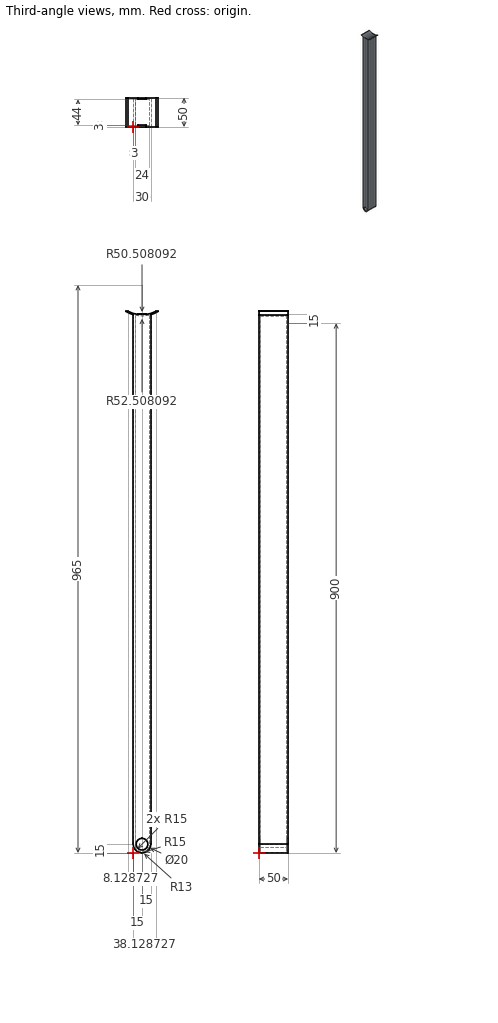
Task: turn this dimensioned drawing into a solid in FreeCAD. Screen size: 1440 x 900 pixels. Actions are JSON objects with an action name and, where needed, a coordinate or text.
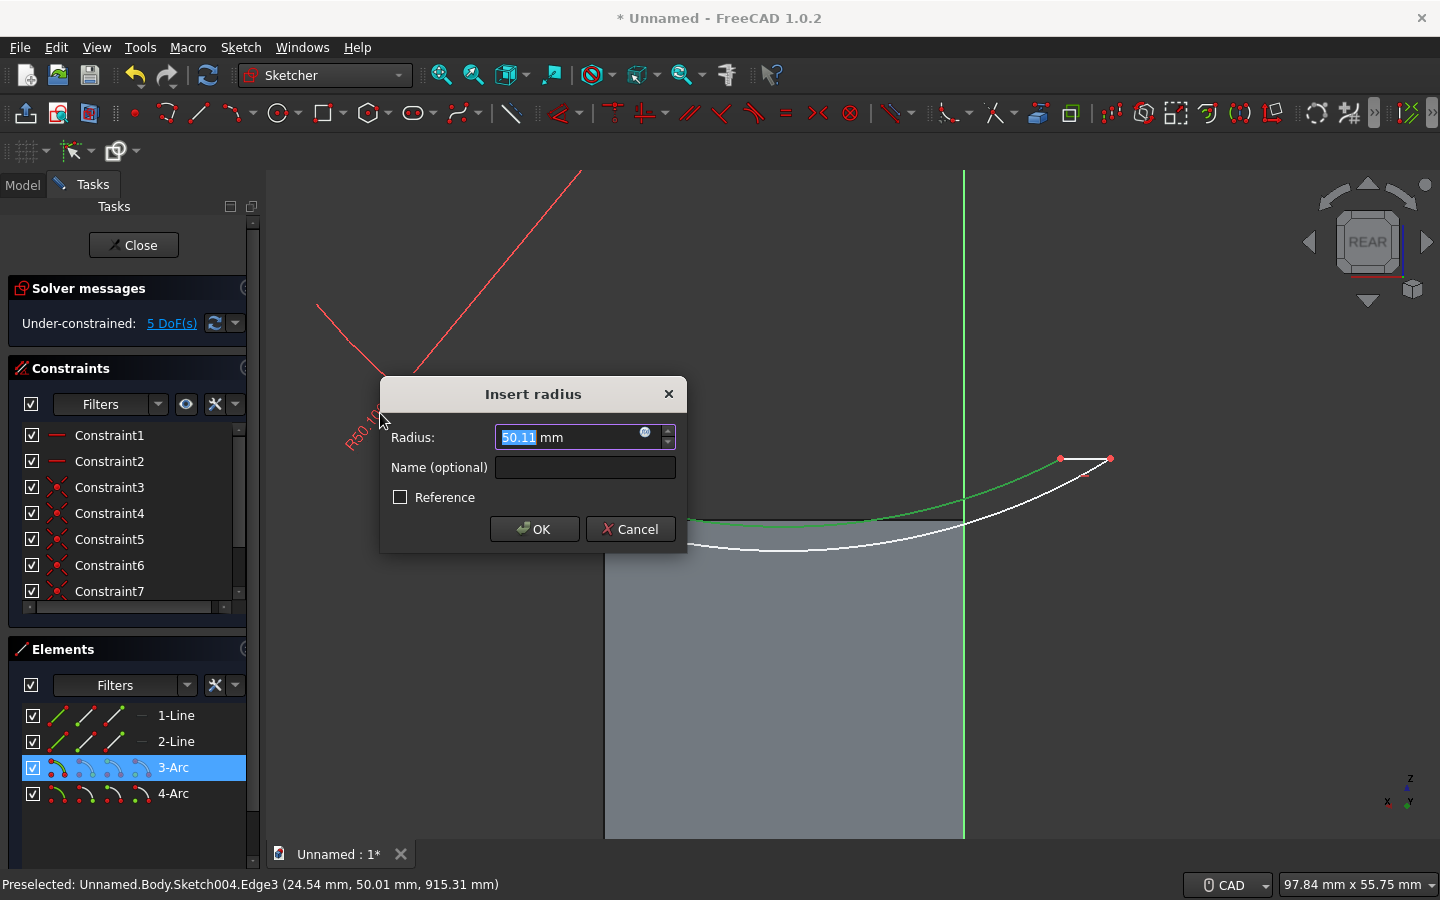
{"action": "type", "text": "50.508092"}
{"action": "key", "text": "Return"}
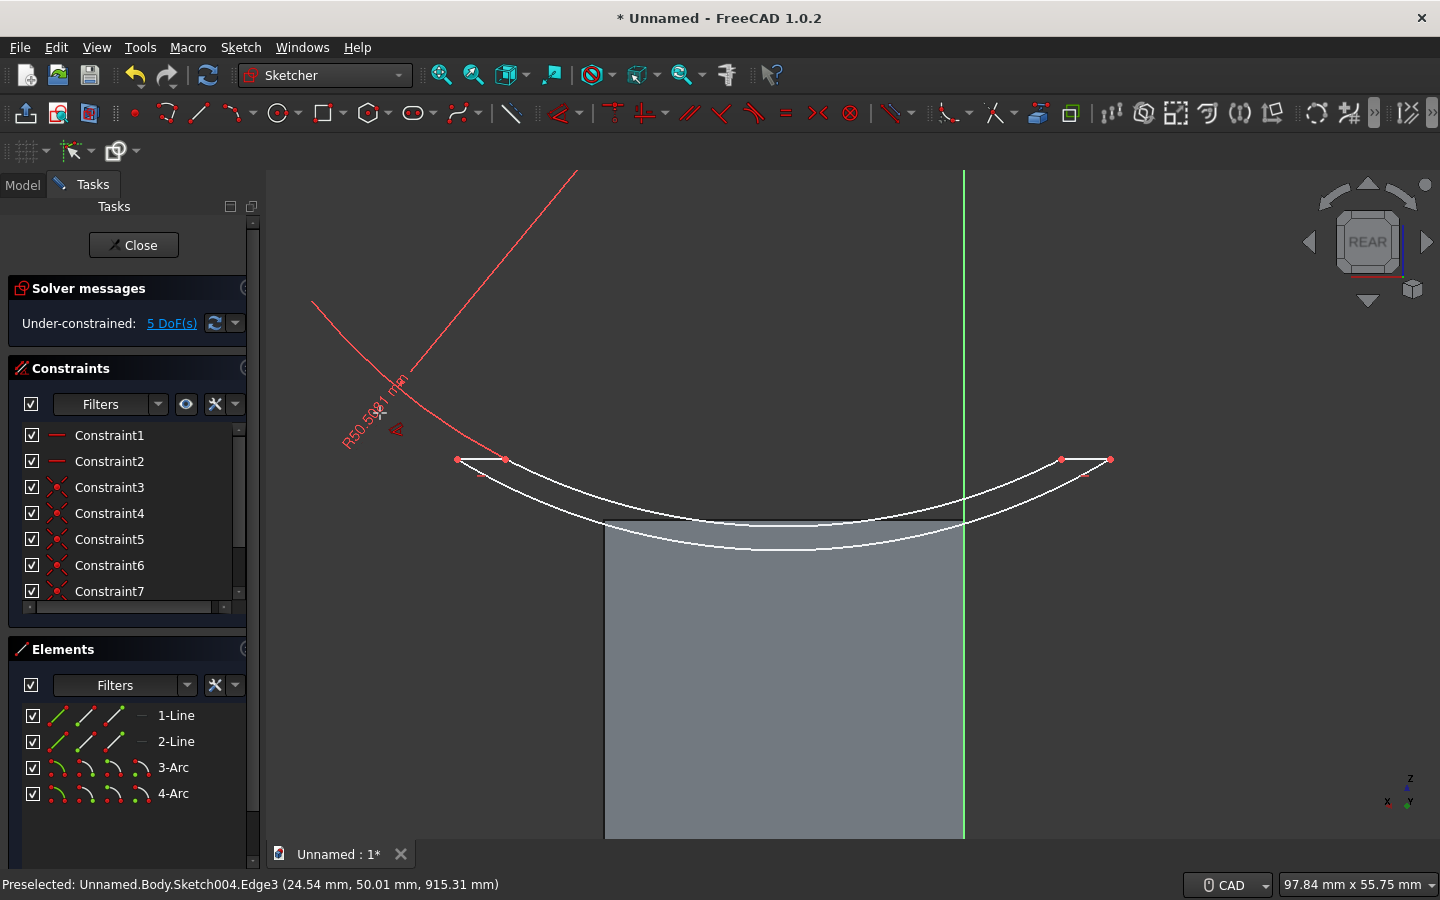
{"action": "left_click", "coordinate": [647, 535]}
{"action": "left_click", "coordinate": [640, 566]}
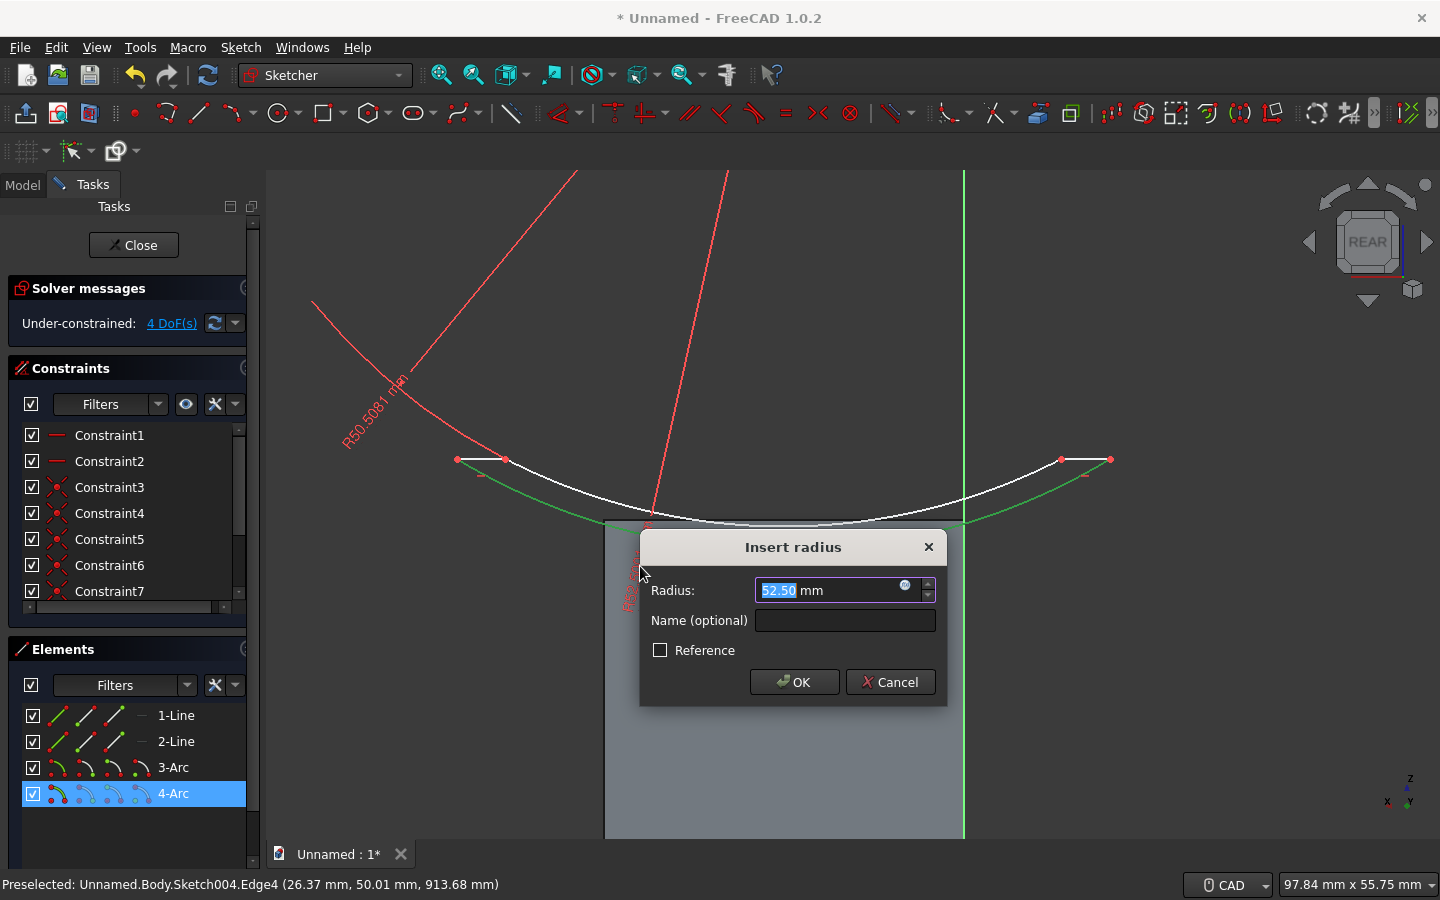
{"action": "type", "text": "52.508092"}
{"action": "key", "text": "Return"}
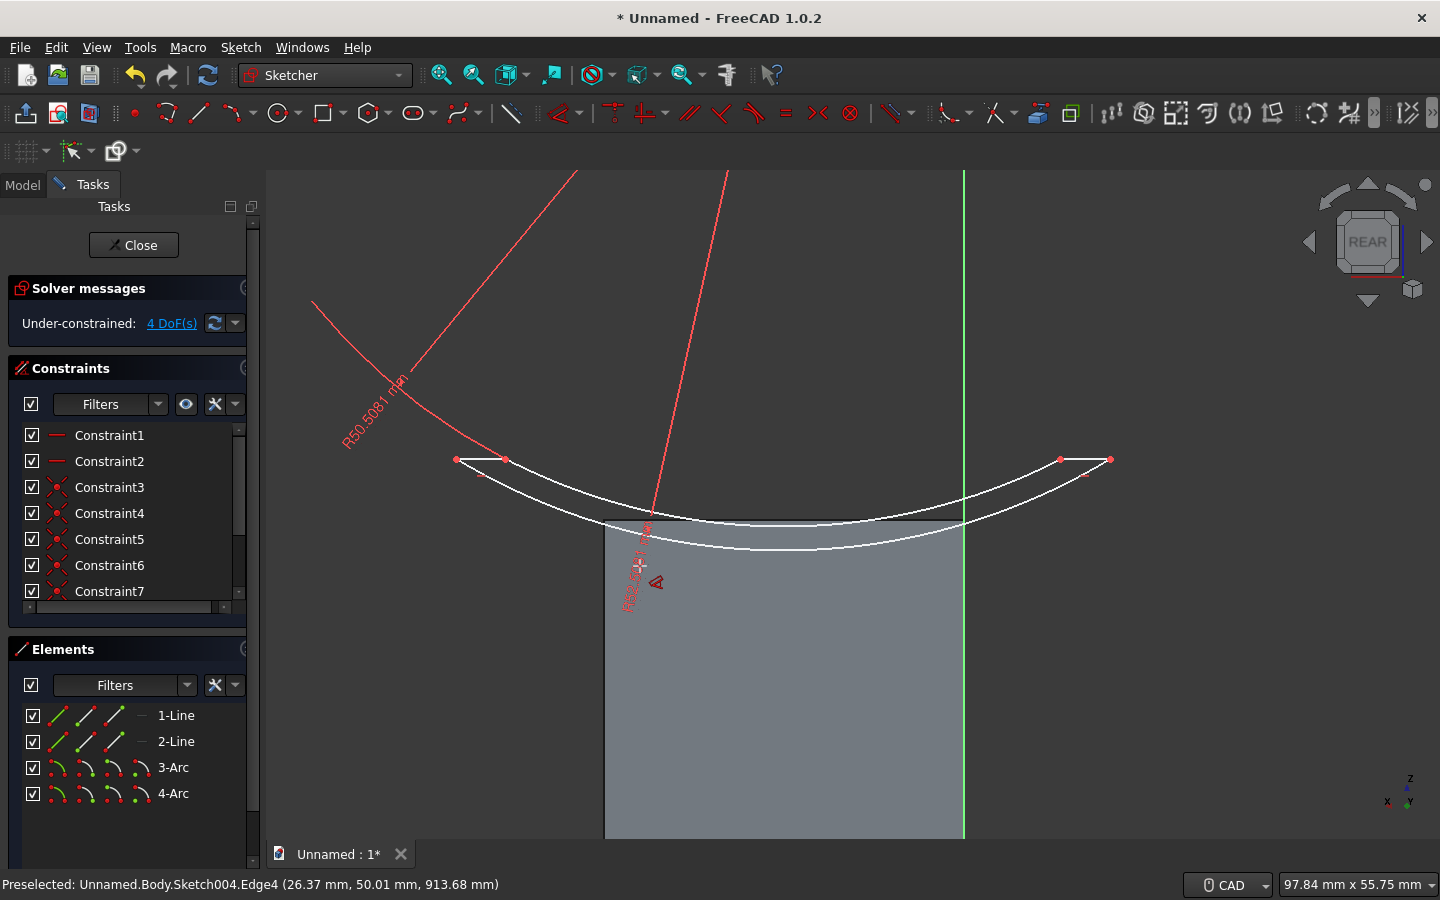
{"action": "scroll", "coordinate": [786, 811], "scroll_direction": "down", "scroll_amount": 3}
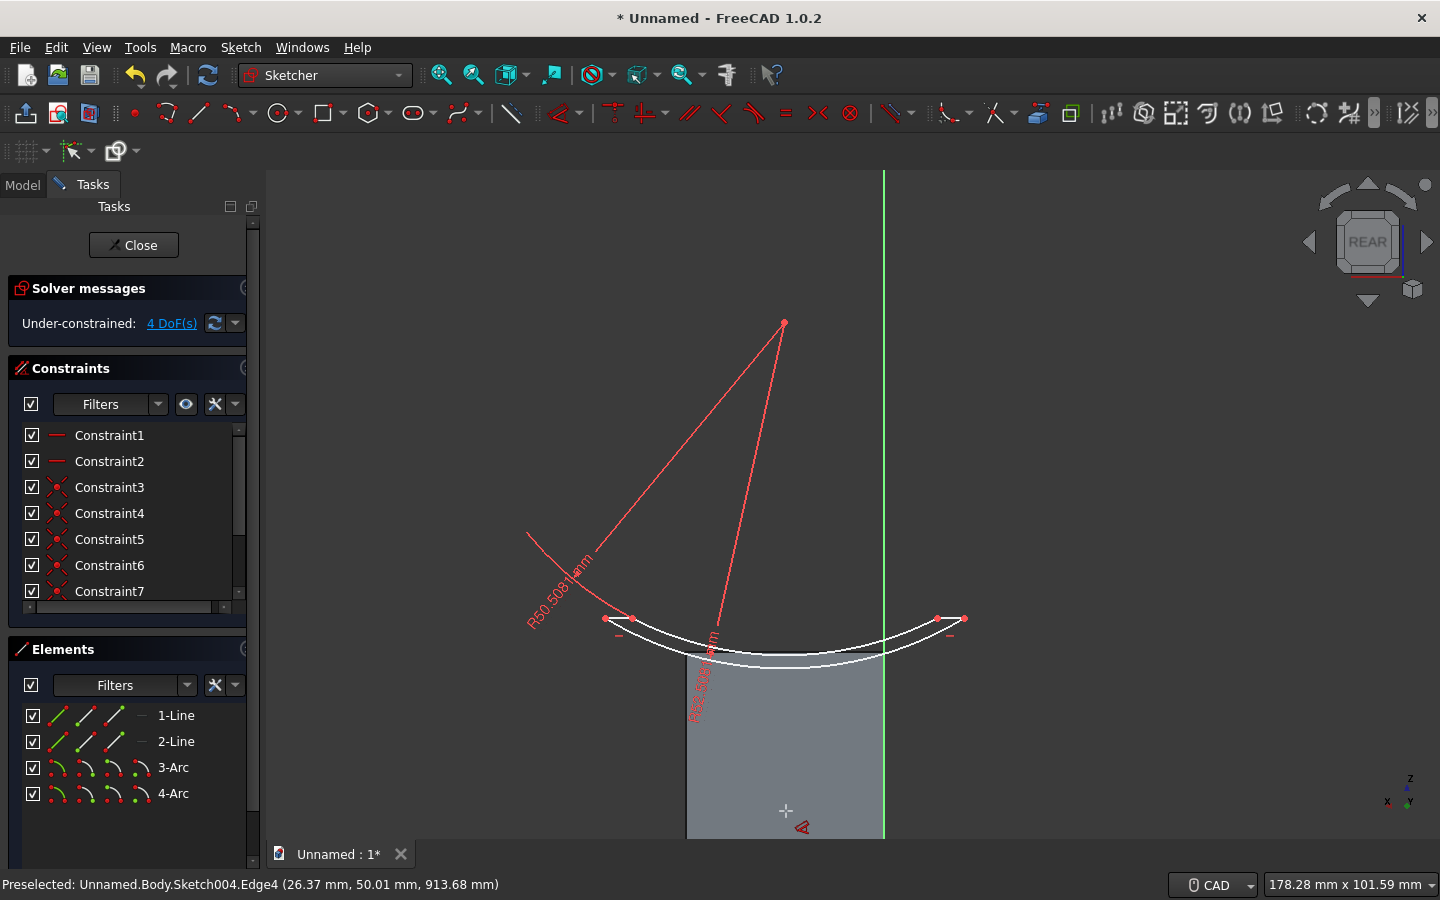
{"action": "left_click", "coordinate": [785, 323]}
{"action": "left_click", "coordinate": [834, 289]}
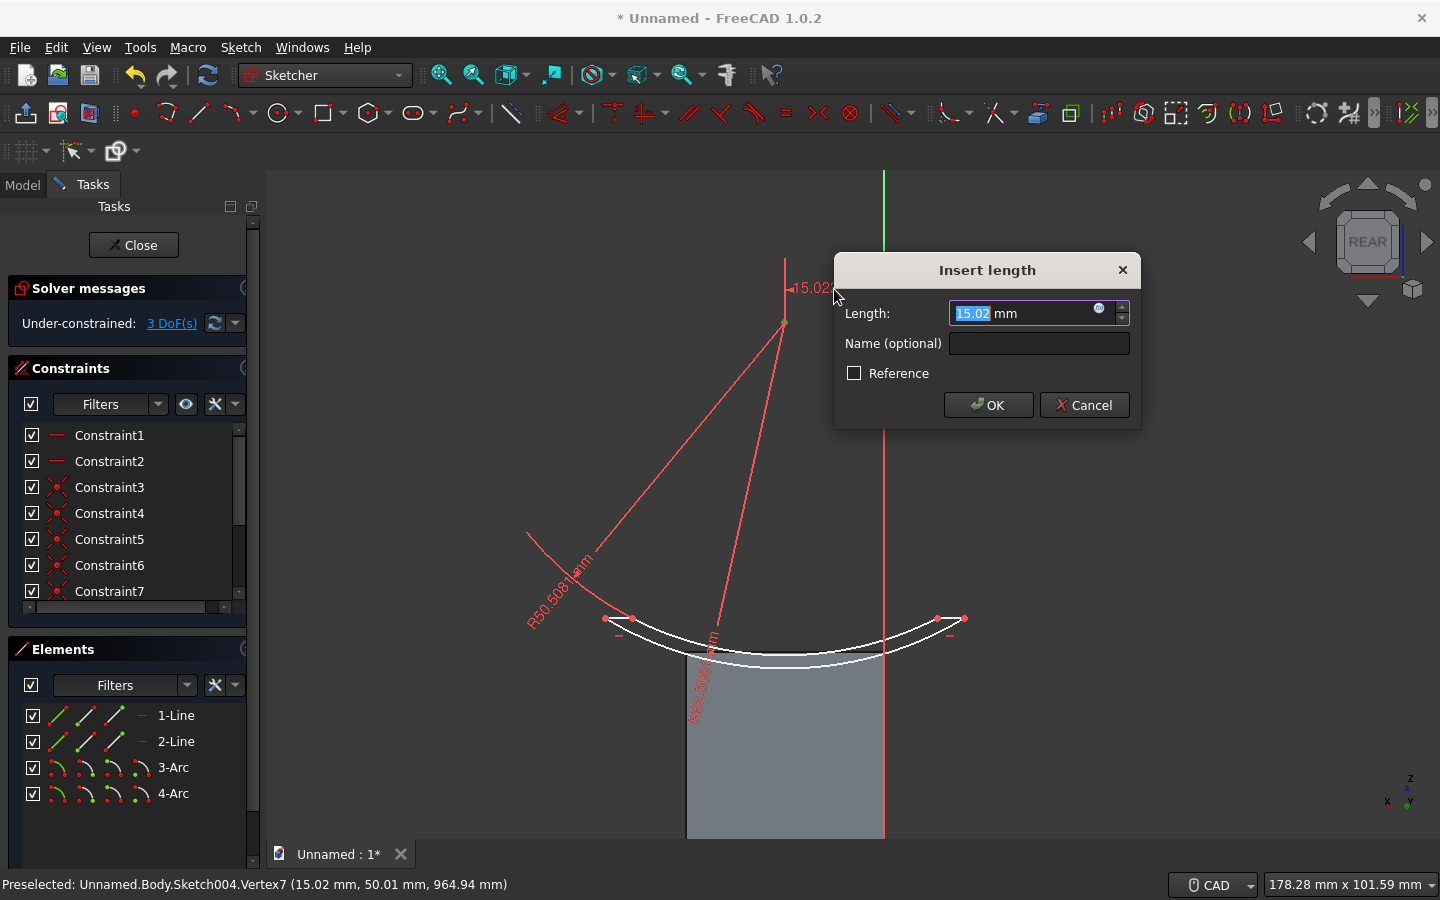
{"action": "type", "text": "15"}
{"action": "key", "text": "Return"}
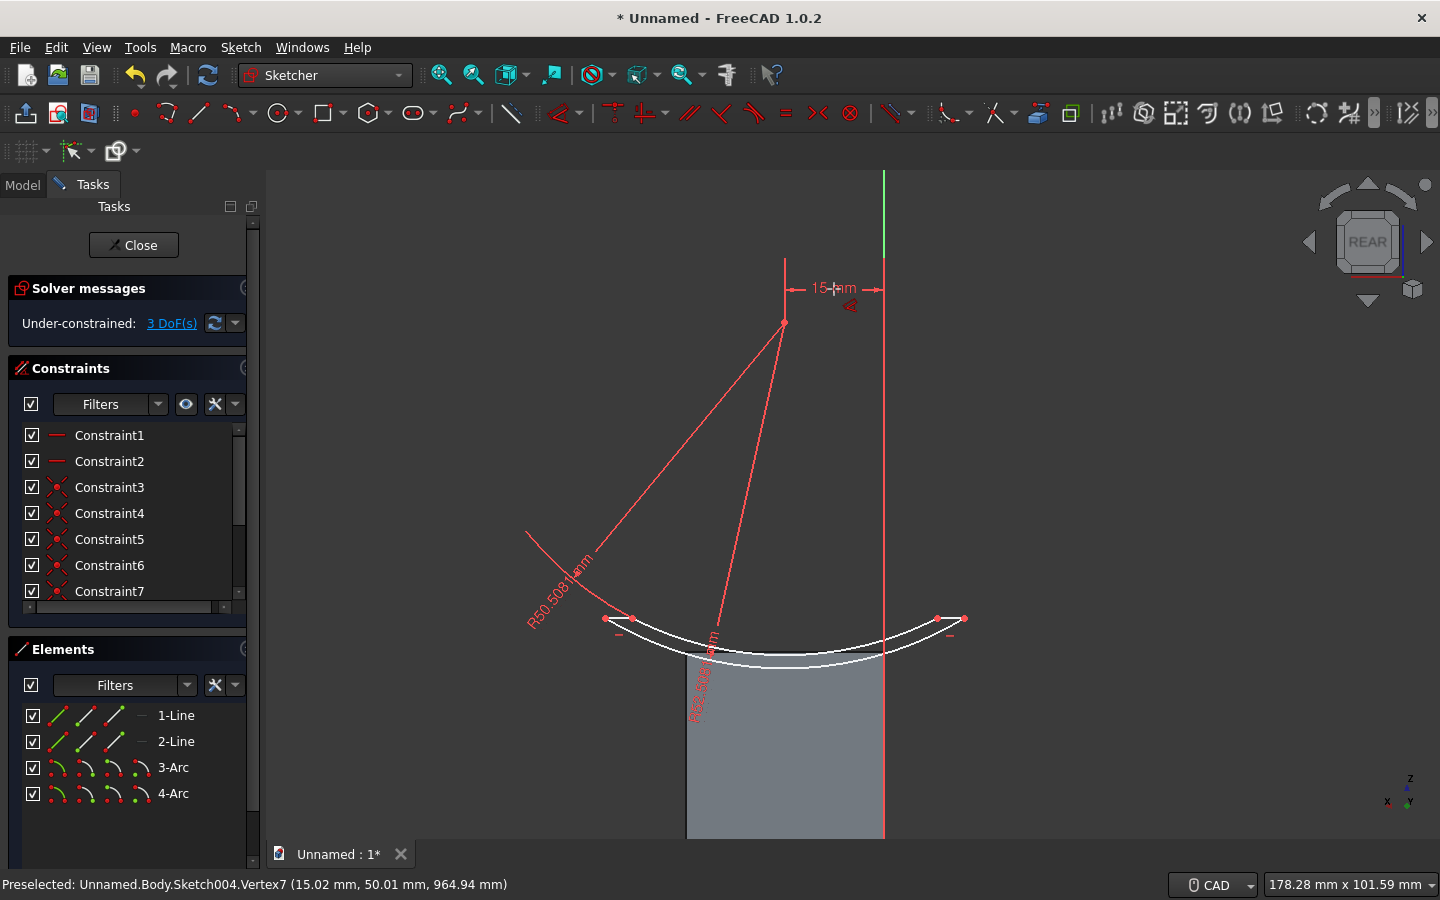
{"action": "left_click", "coordinate": [785, 323]}
{"action": "left_click", "coordinate": [918, 567]}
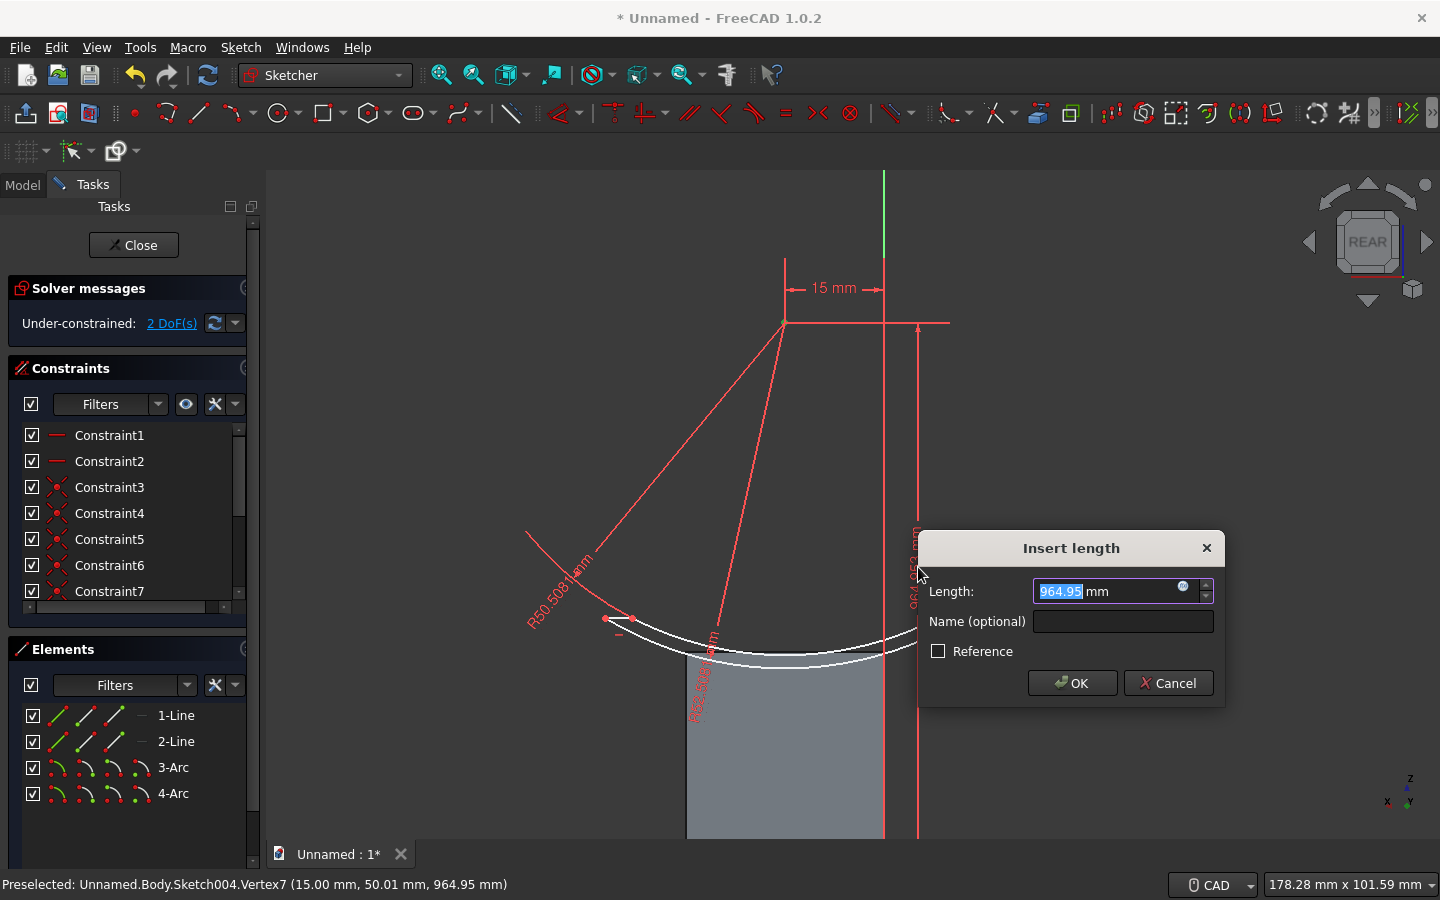
{"action": "type", "text": "965"}
{"action": "key", "text": "Return"}